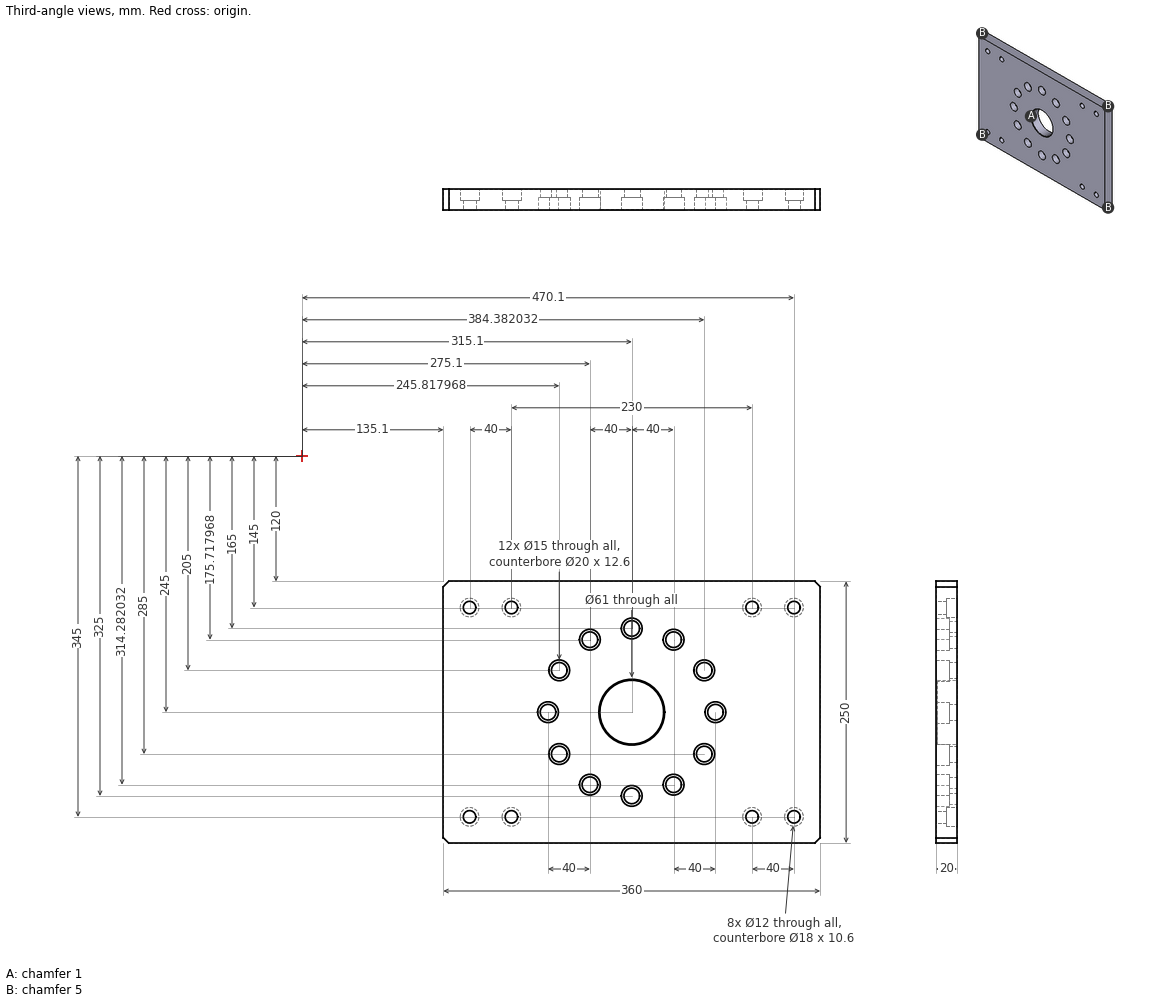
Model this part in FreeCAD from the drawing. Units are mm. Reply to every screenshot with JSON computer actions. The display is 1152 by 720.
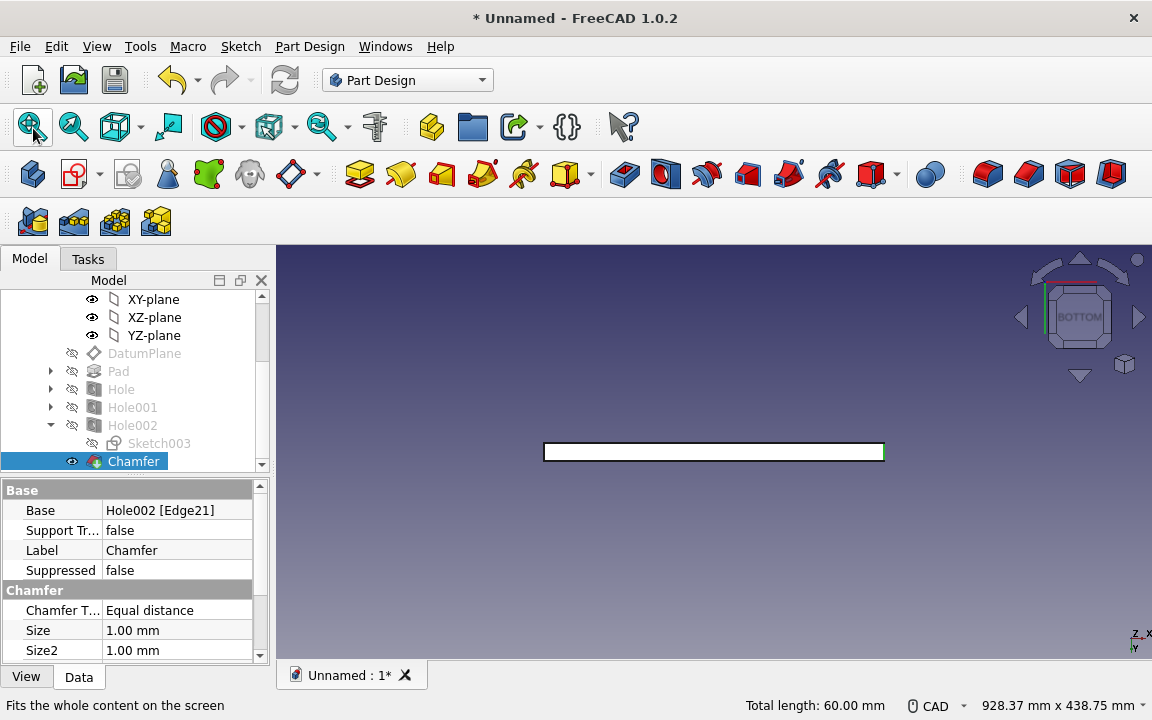
{"action": "left_click", "coordinate": [544, 451], "text": "ctrl"}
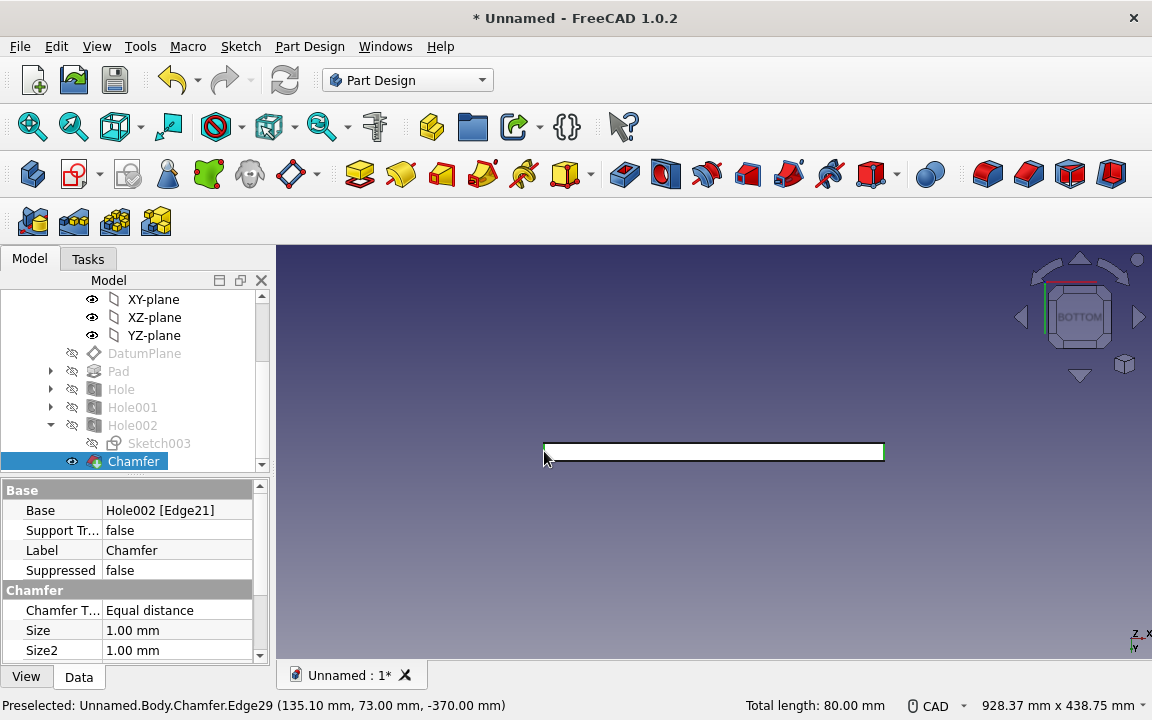
{"action": "left_click", "coordinate": [1029, 174]}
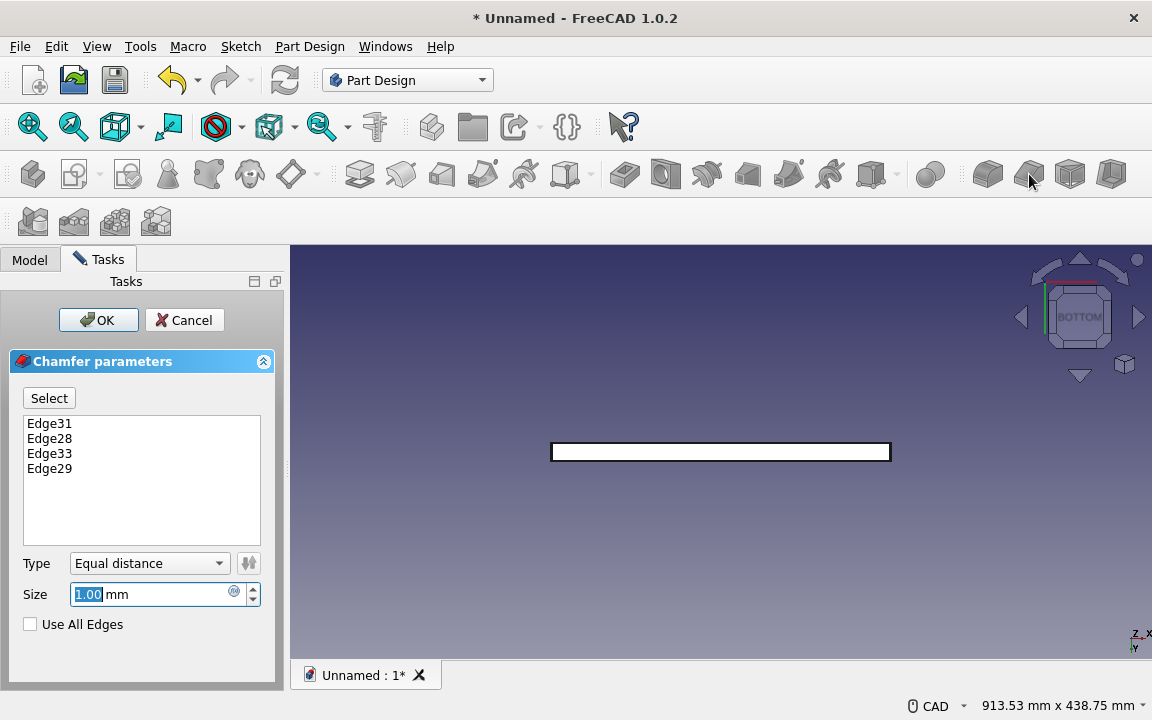
{"action": "type", "text": "5"}
{"action": "key", "text": "Tab"}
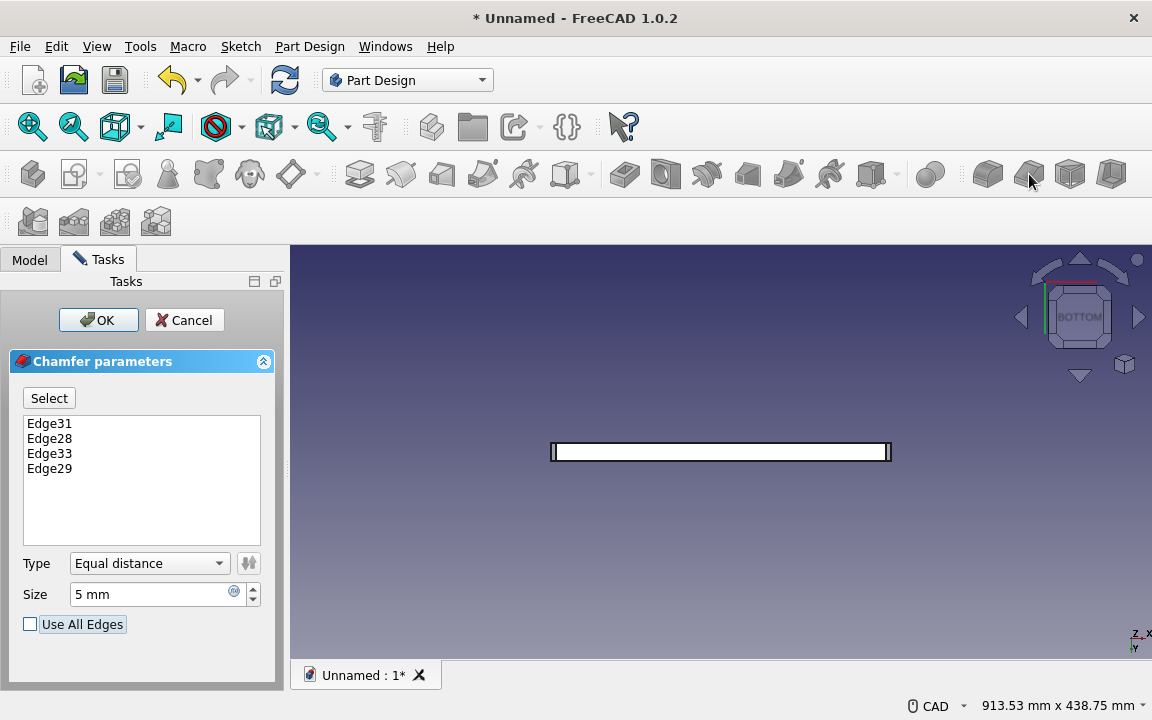
{"action": "left_click", "coordinate": [99, 320]}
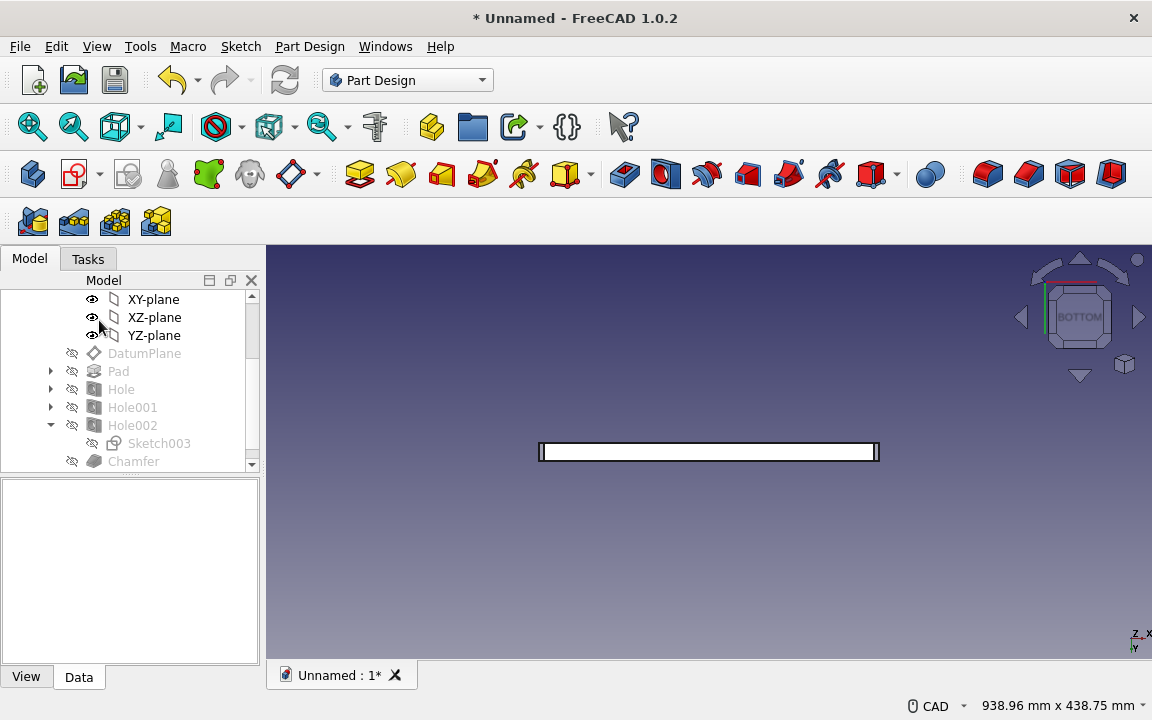
{"action": "key", "text": "0"}